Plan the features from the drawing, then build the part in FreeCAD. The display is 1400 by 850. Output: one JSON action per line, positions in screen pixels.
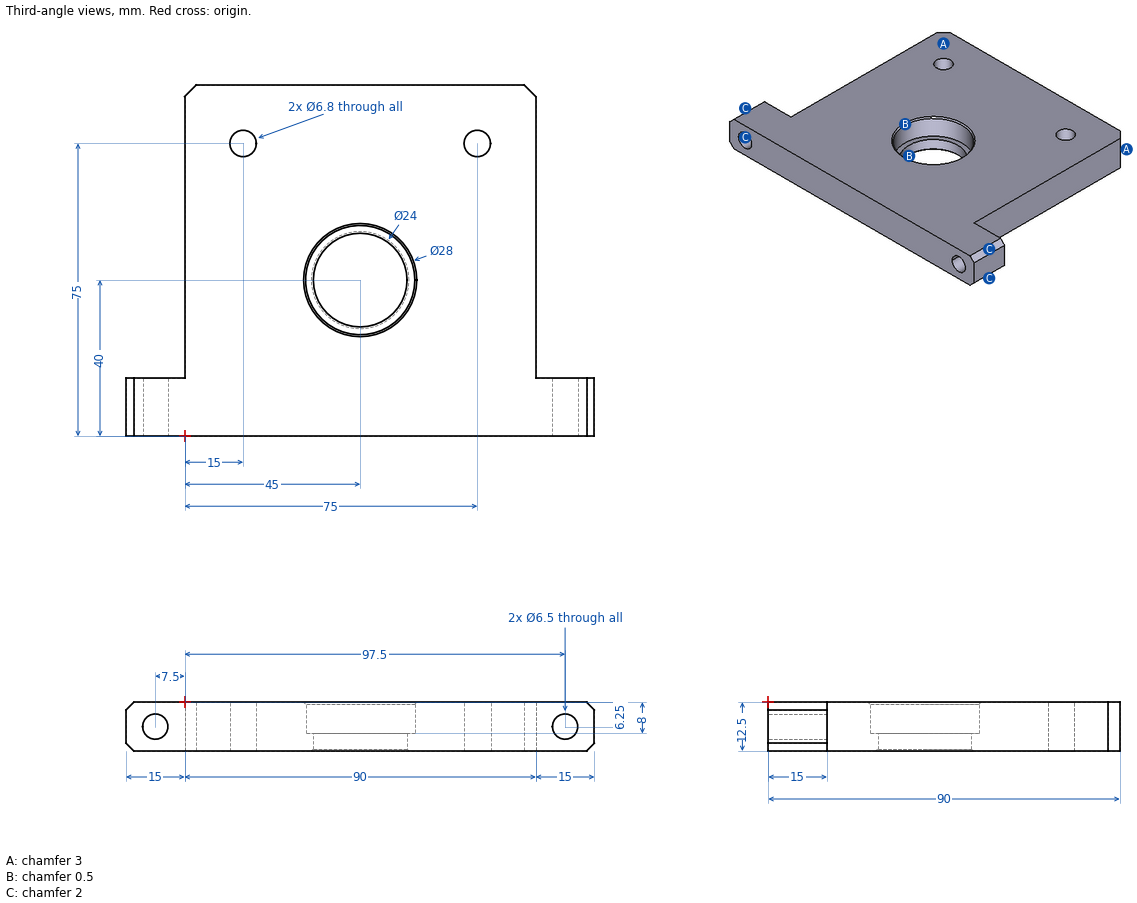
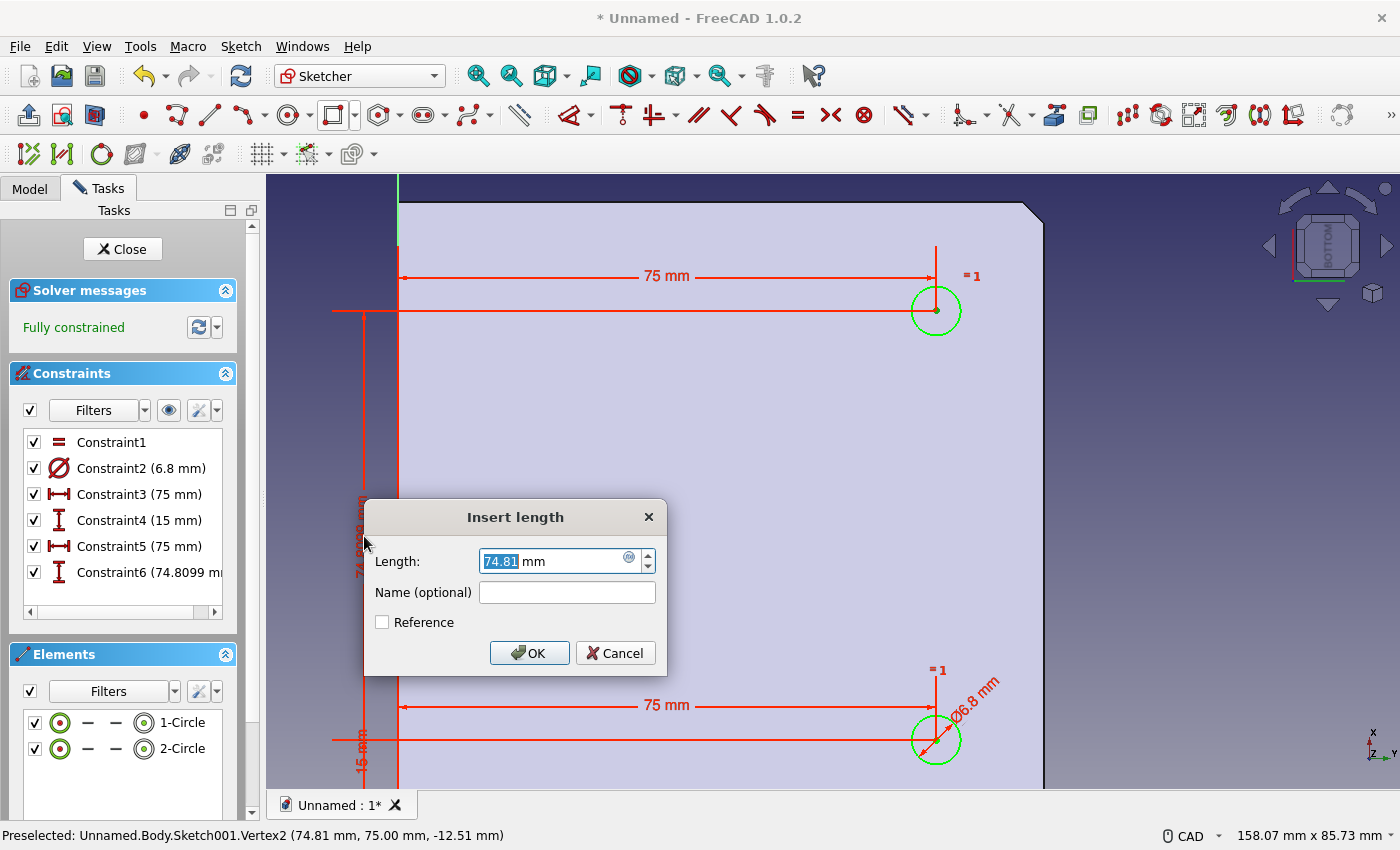
{"action": "type", "text": "75"}
{"action": "key", "text": "Return"}
{"action": "key", "text": "Escape"}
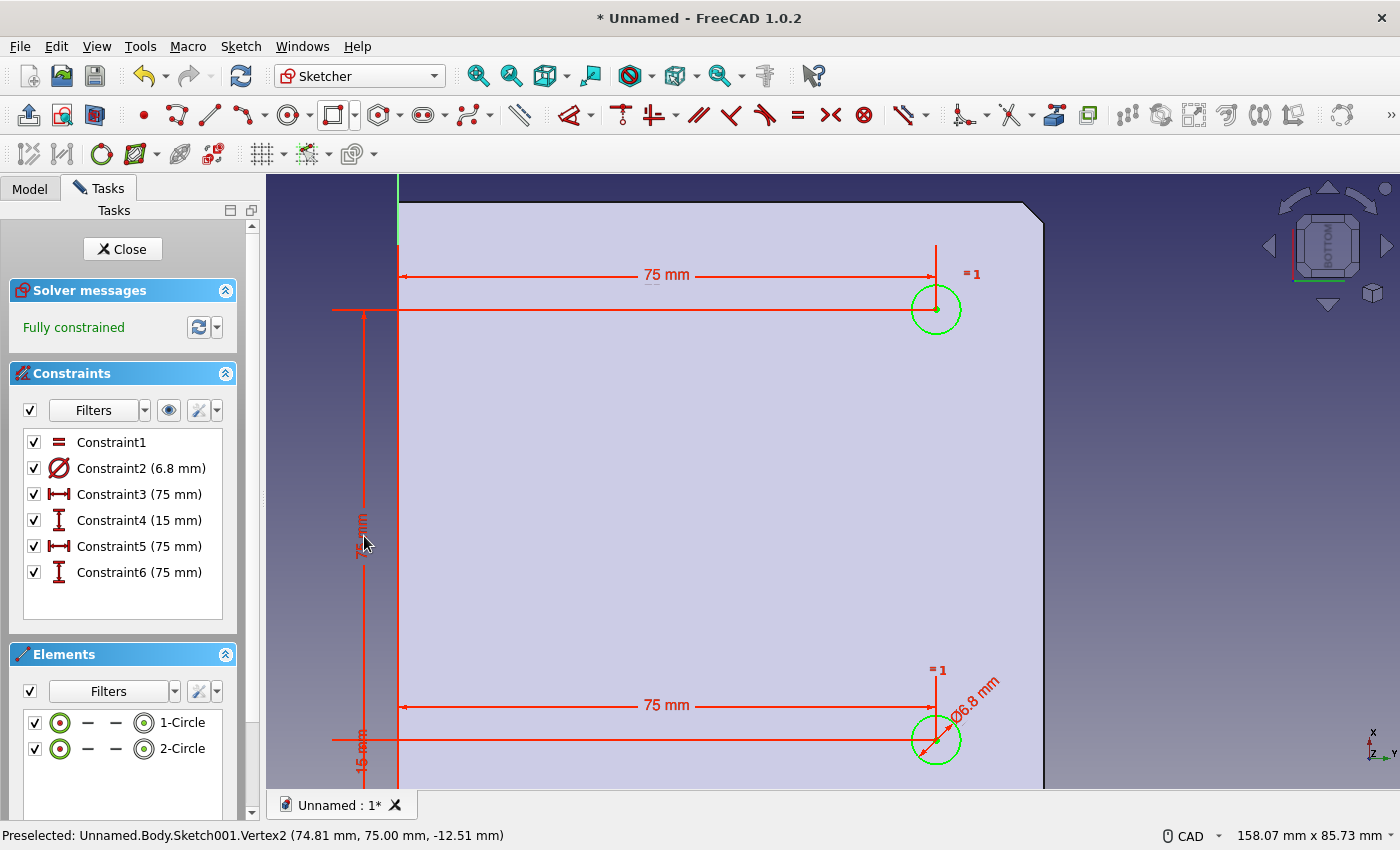
{"action": "left_click", "coordinate": [123, 249]}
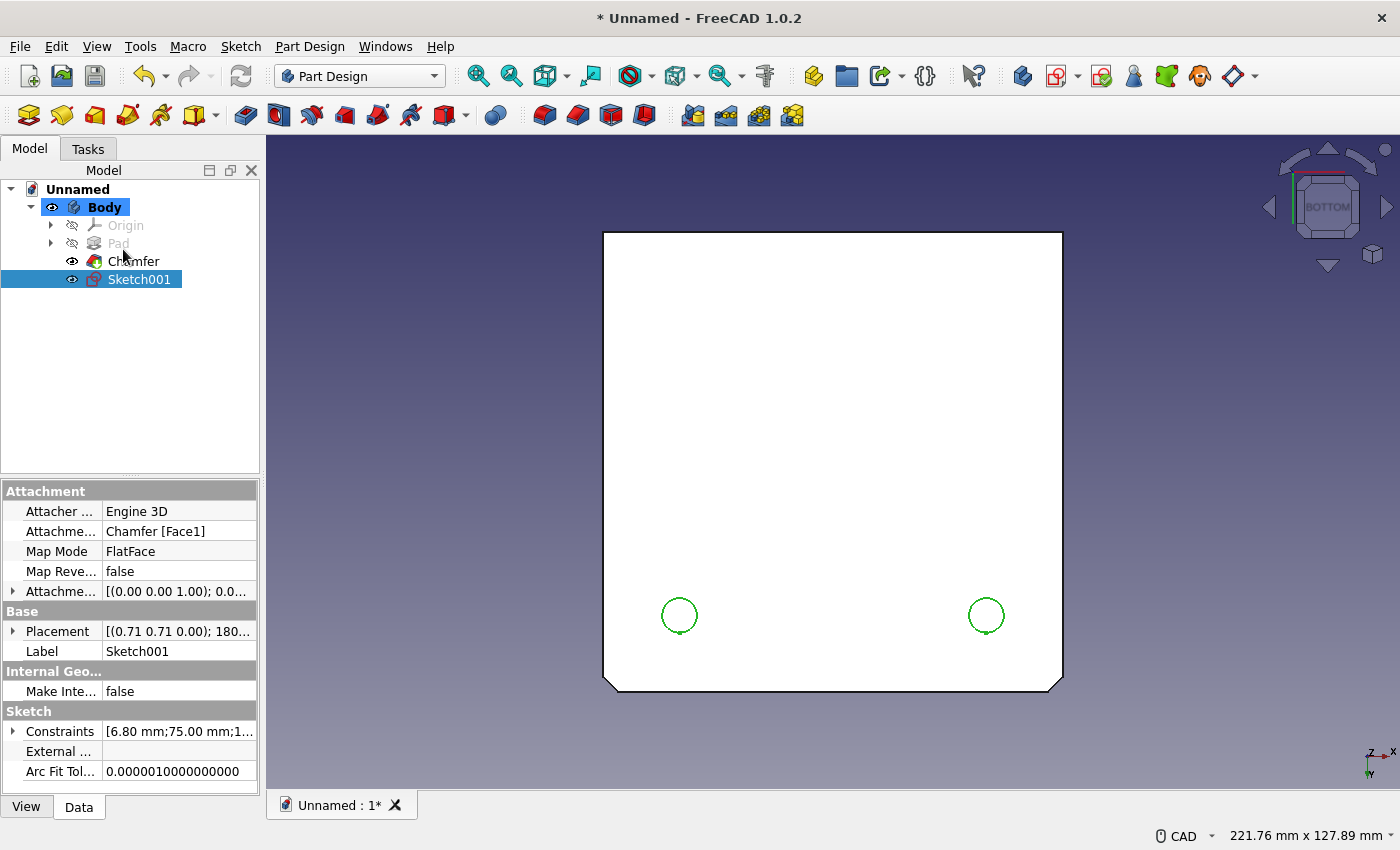
{"action": "left_click", "coordinate": [279, 116]}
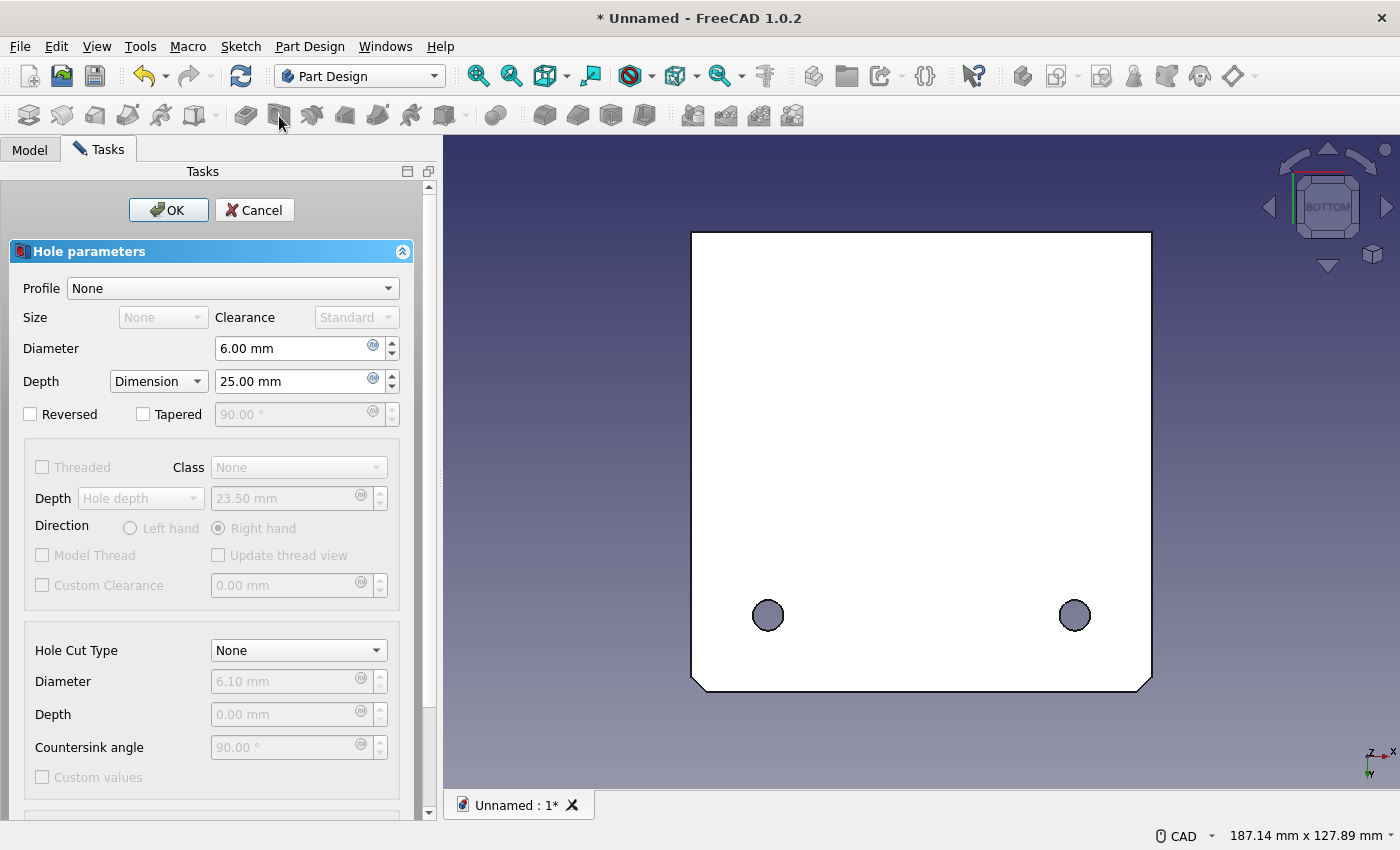
{"action": "triple_click", "coordinate": [300, 348]}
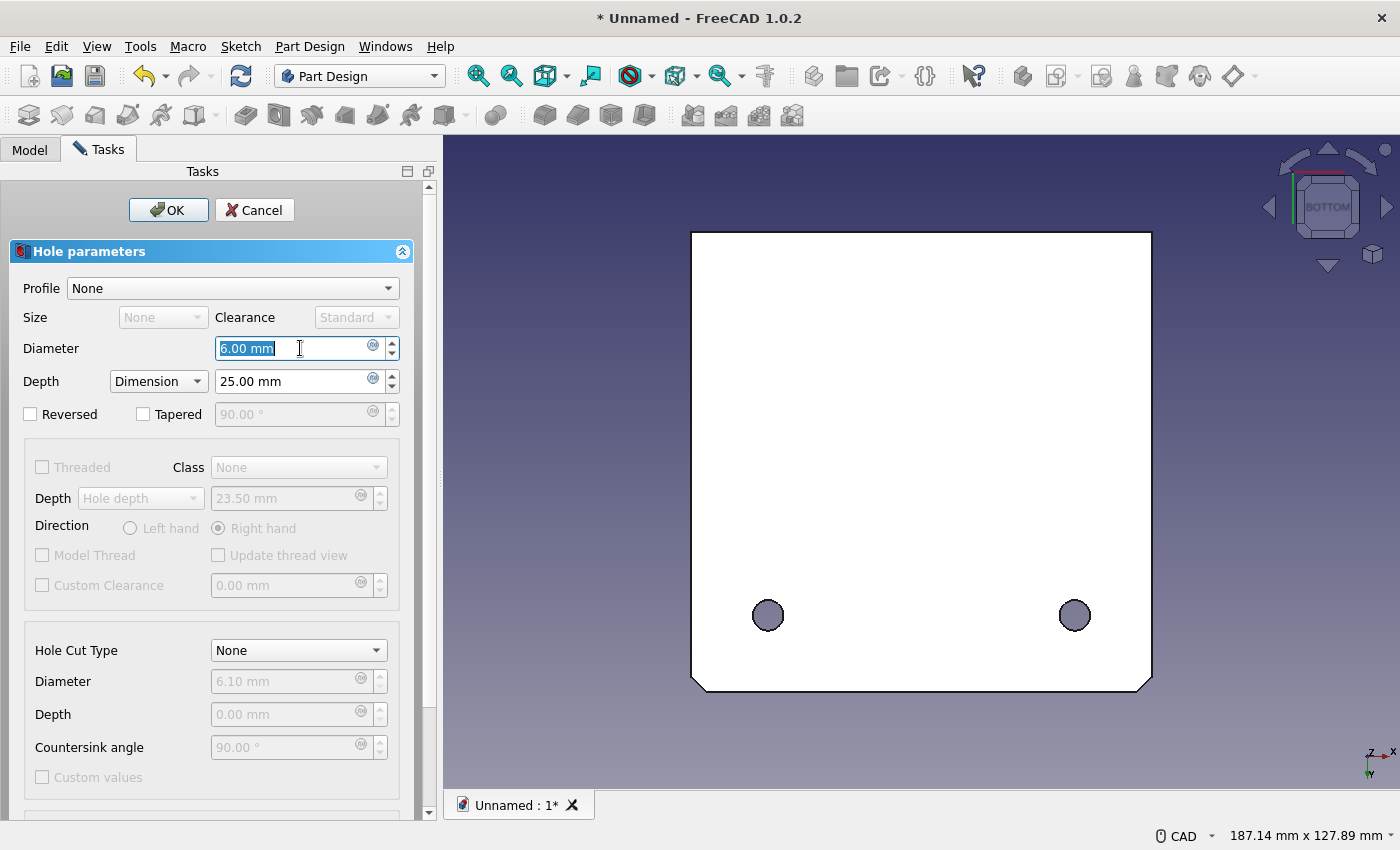
{"action": "type", "text": "6.8"}
{"action": "key", "text": "Tab"}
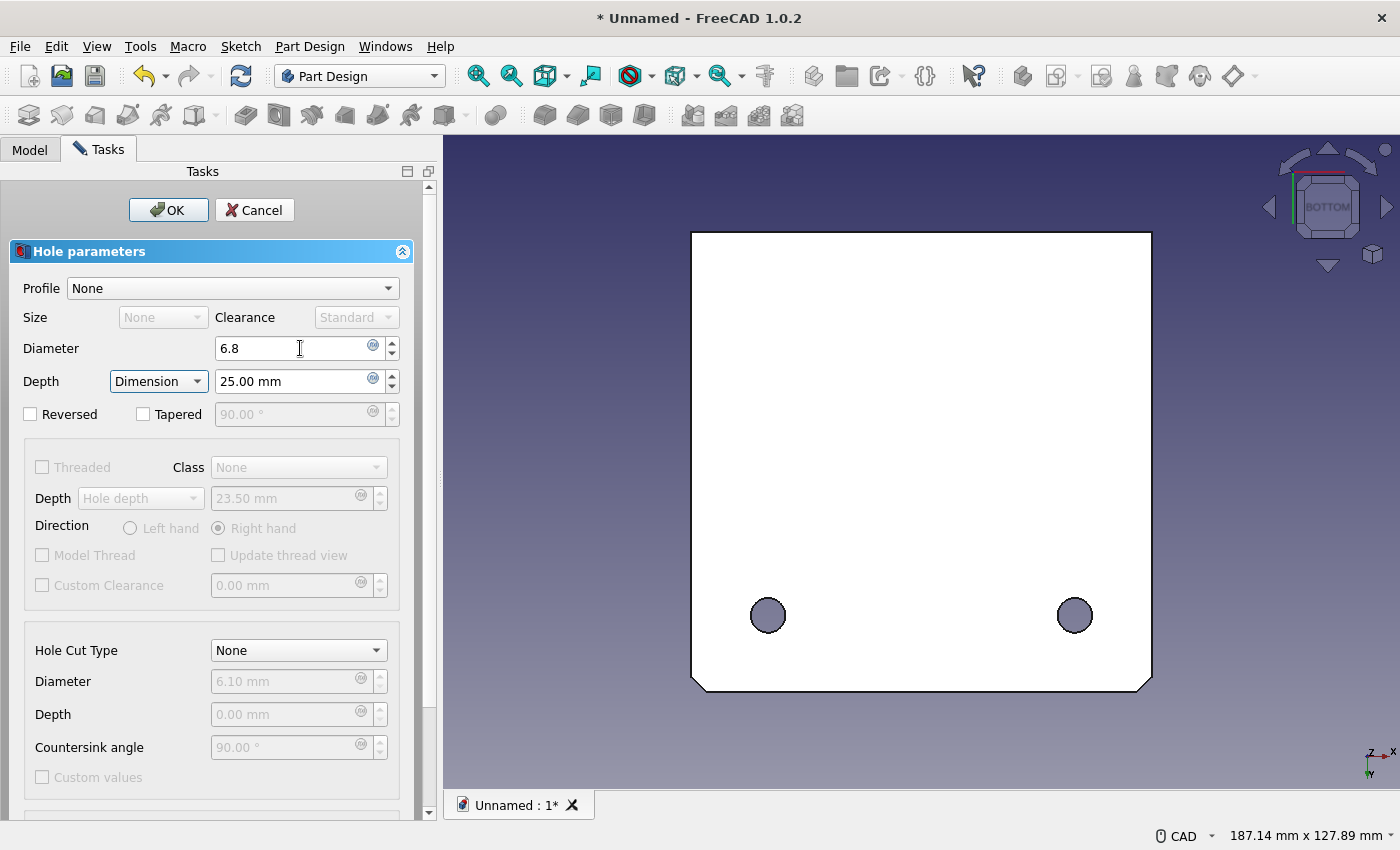
{"action": "left_click", "coordinate": [160, 382]}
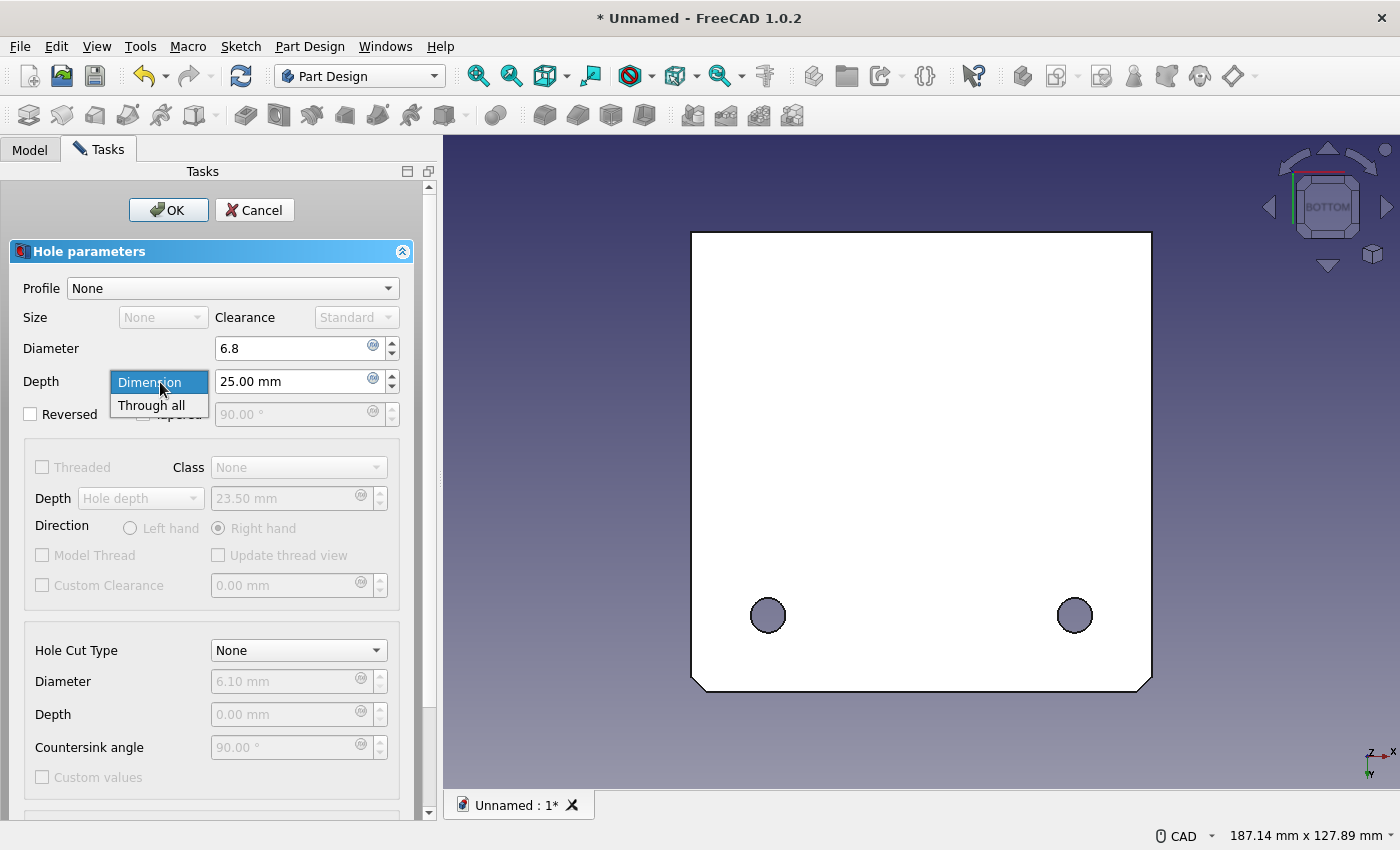
{"action": "left_click", "coordinate": [158, 406]}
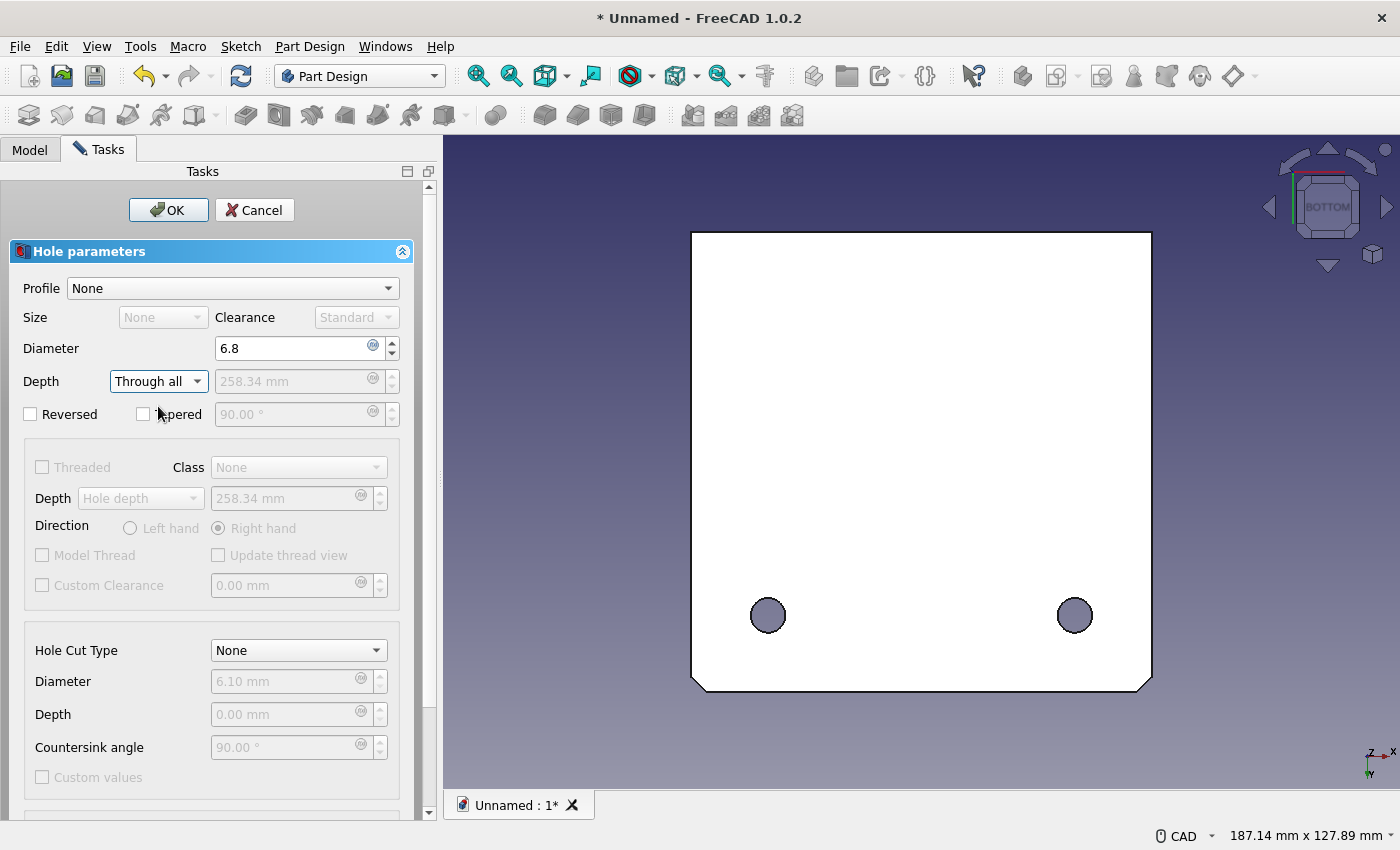
{"action": "left_click", "coordinate": [169, 210]}